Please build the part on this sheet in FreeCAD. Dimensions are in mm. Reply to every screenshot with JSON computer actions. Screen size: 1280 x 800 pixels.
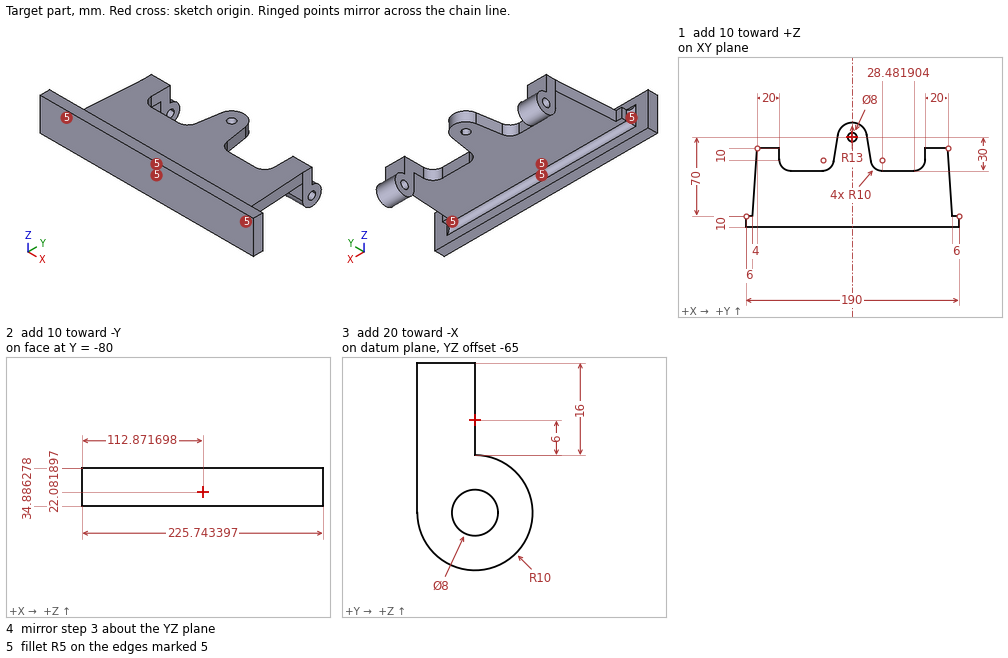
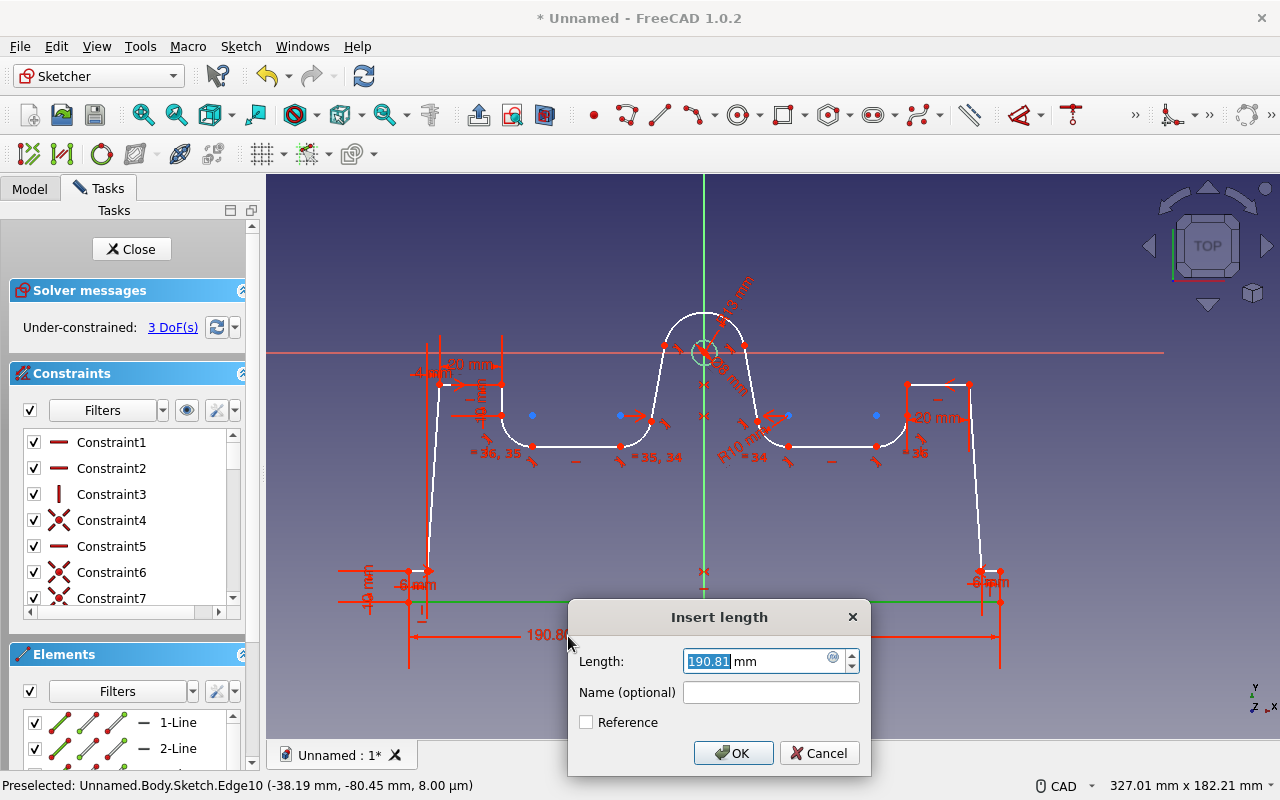
{"action": "type", "text": "190"}
{"action": "key", "text": "Return"}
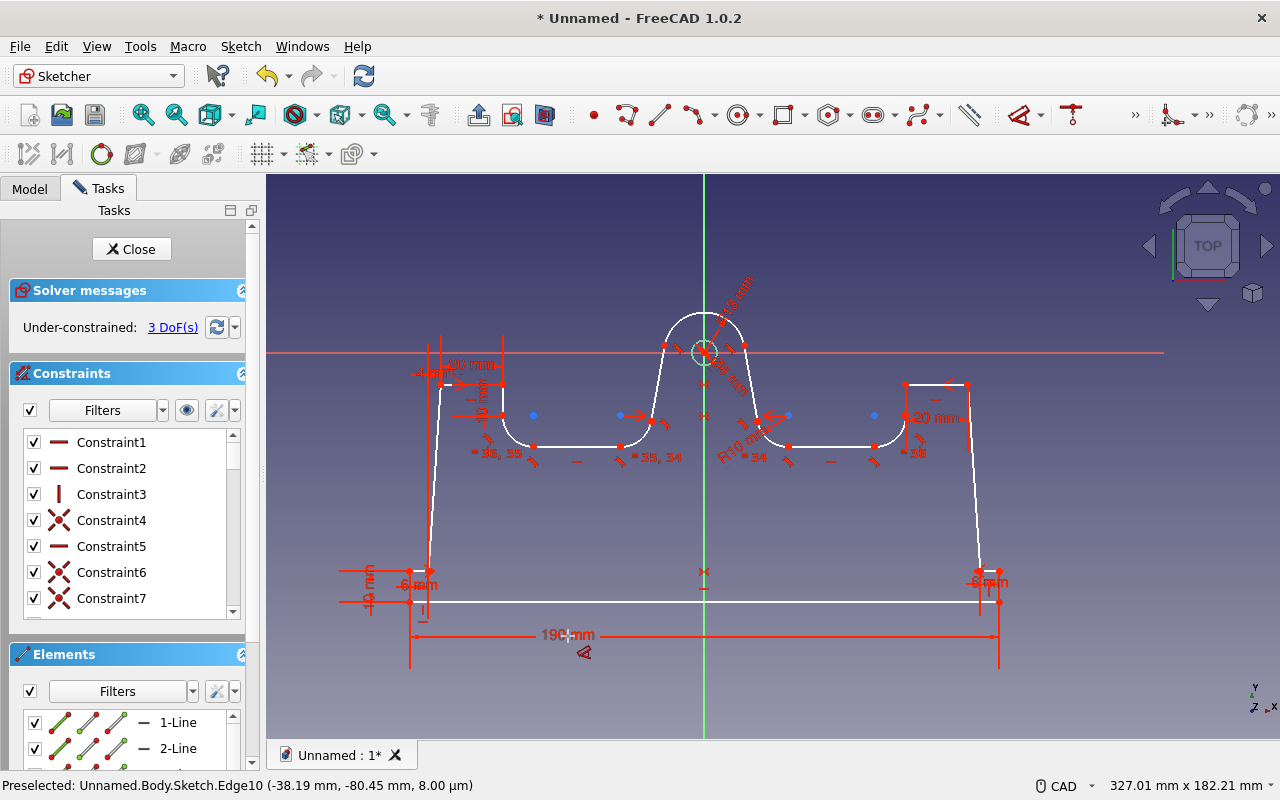
{"action": "left_click", "coordinate": [875, 447]}
{"action": "left_click", "coordinate": [909, 367]}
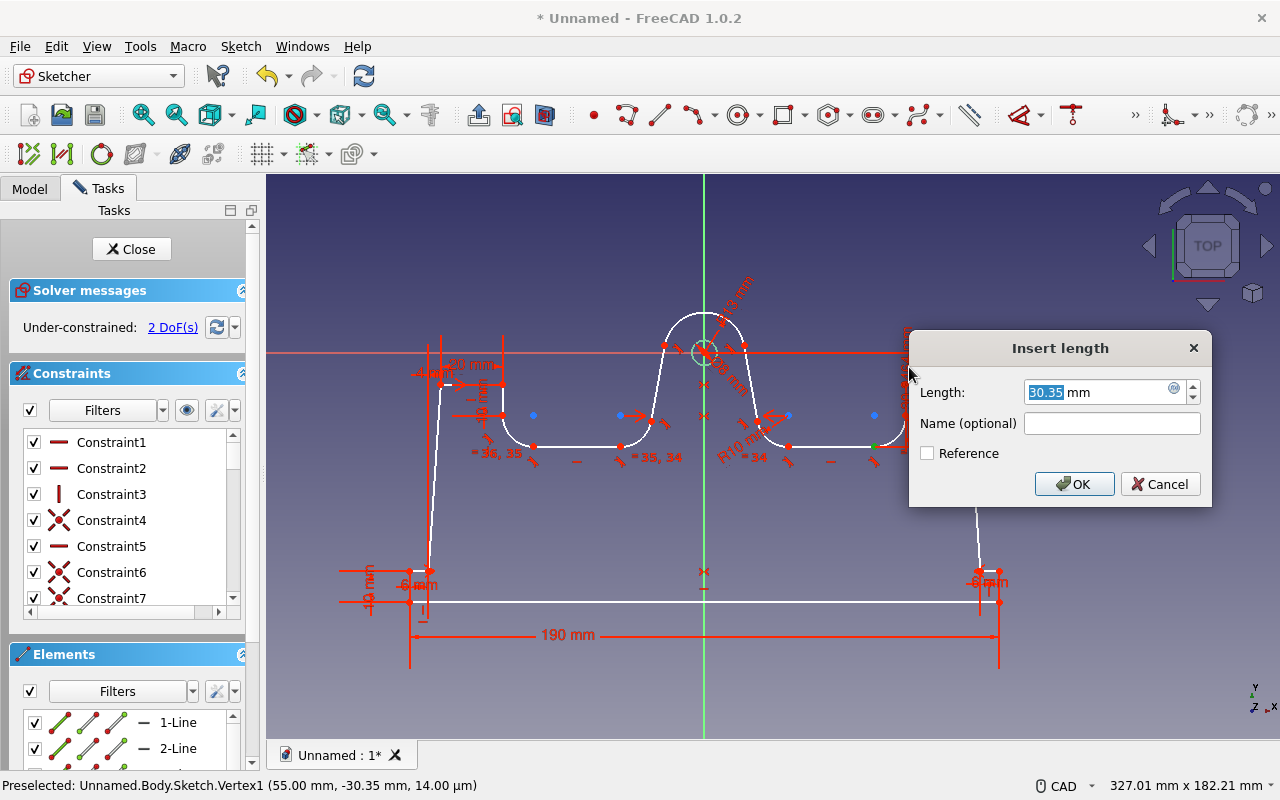
{"action": "type", "text": "30"}
{"action": "key", "text": "Return"}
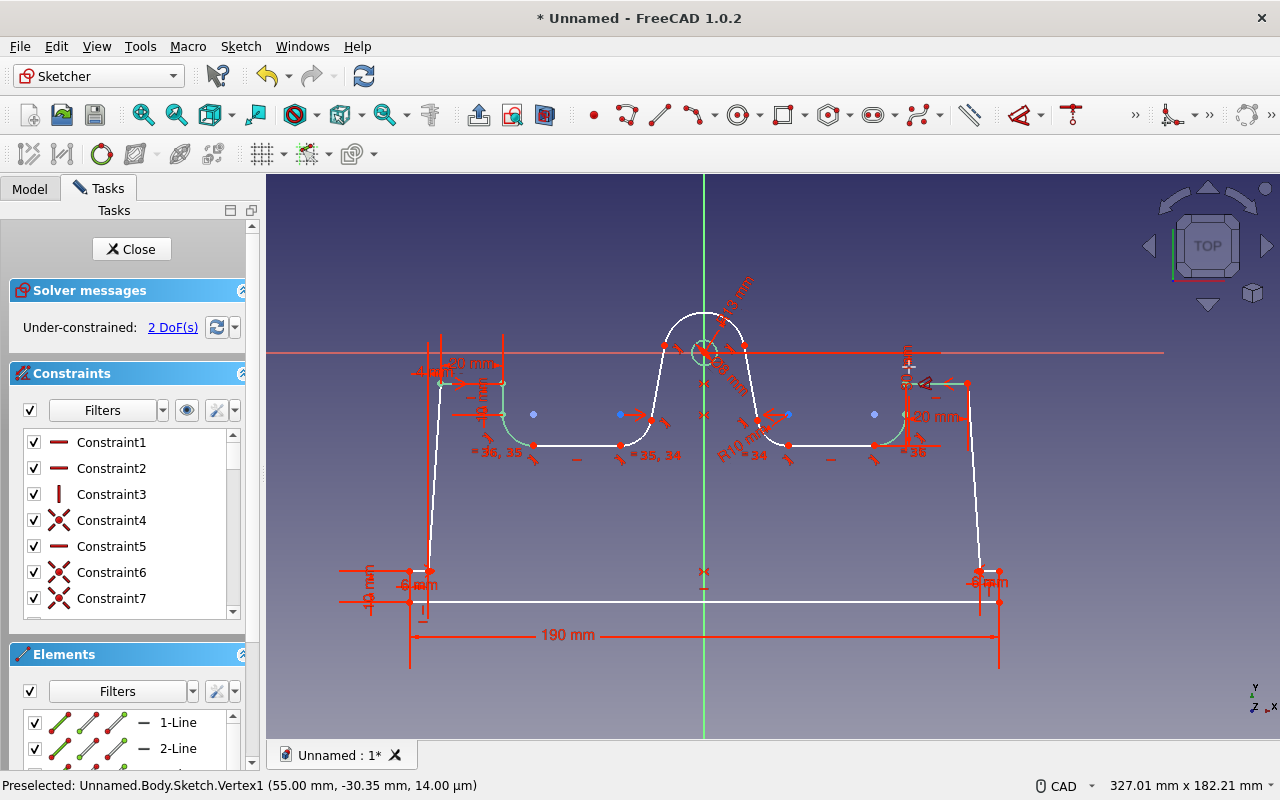
{"action": "left_click", "coordinate": [428, 571]}
{"action": "left_click", "coordinate": [394, 462]}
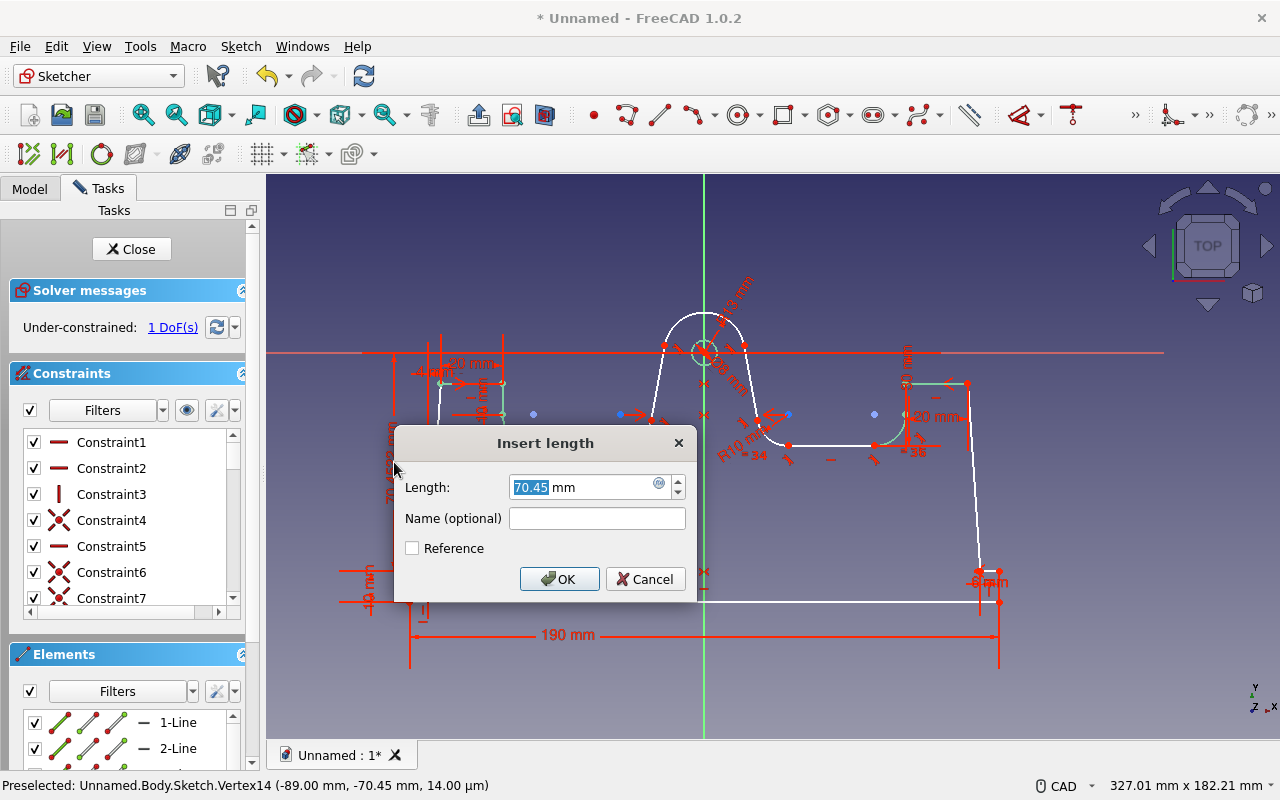
{"action": "type", "text": "70"}
{"action": "key", "text": "Return"}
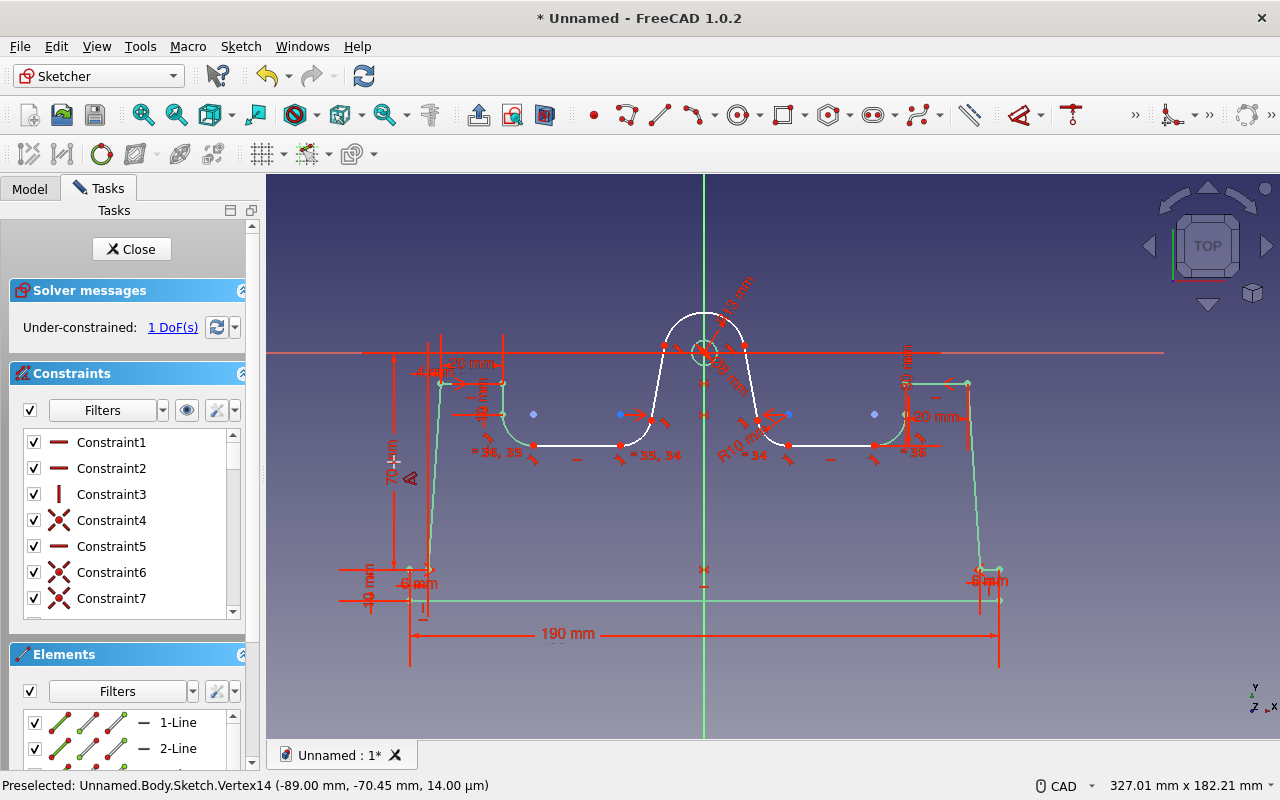
{"action": "left_click", "coordinate": [849, 446]}
{"action": "left_click", "coordinate": [832, 412]}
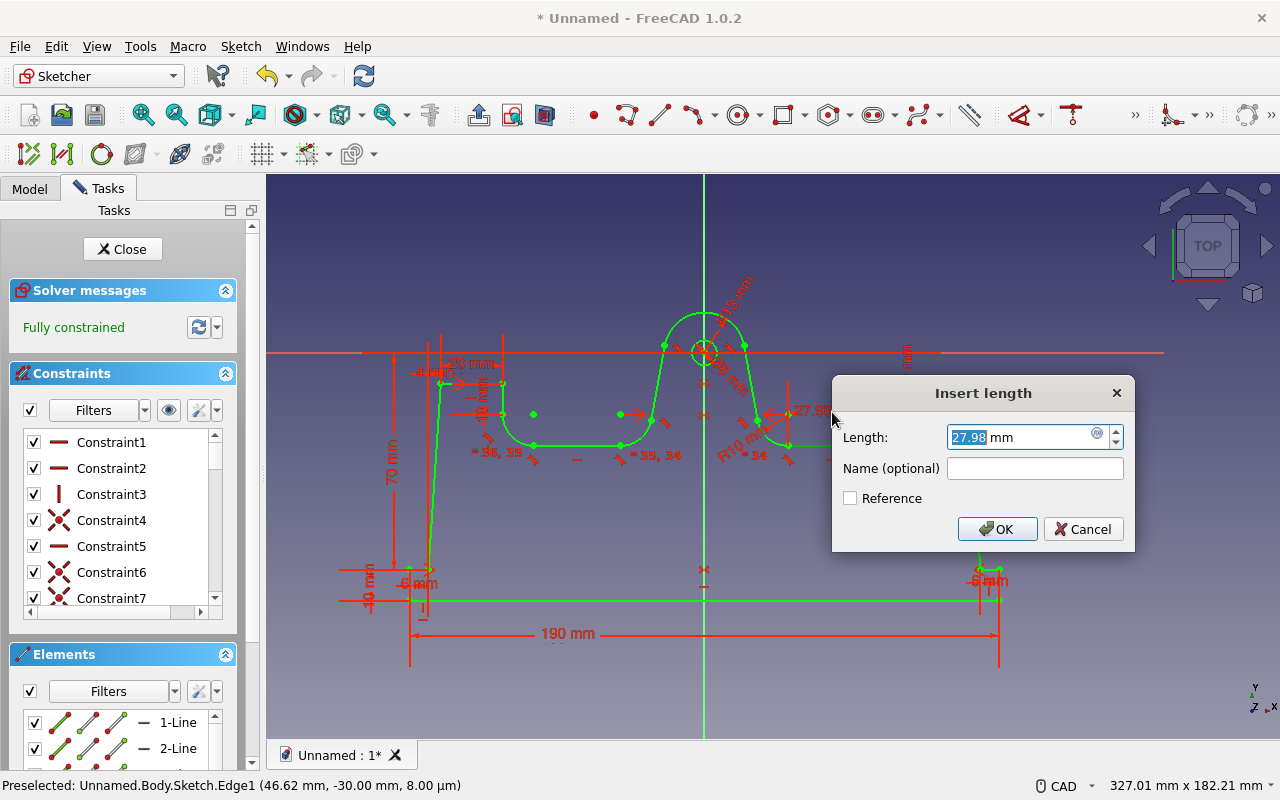
{"action": "type", "text": "28.481904"}
{"action": "key", "text": "Return"}
{"action": "key", "text": "Escape"}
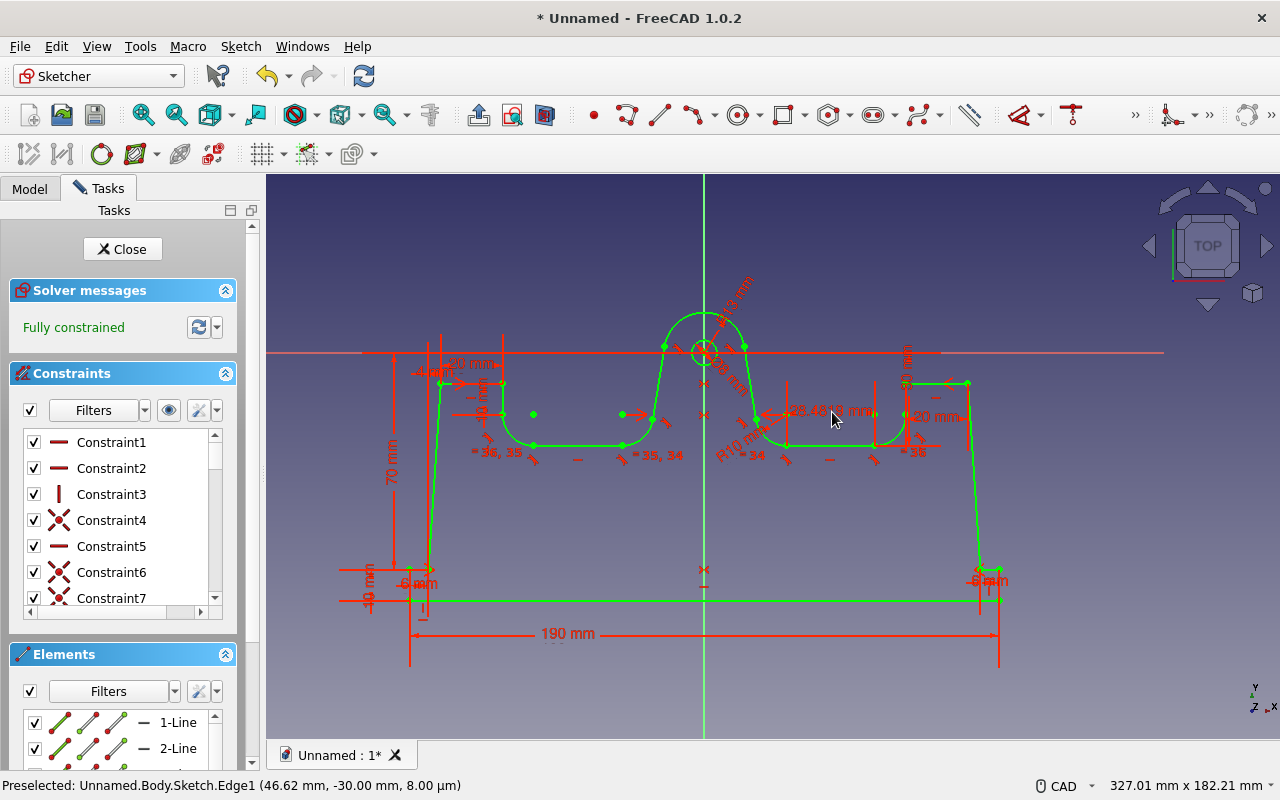
{"action": "left_click", "coordinate": [123, 249]}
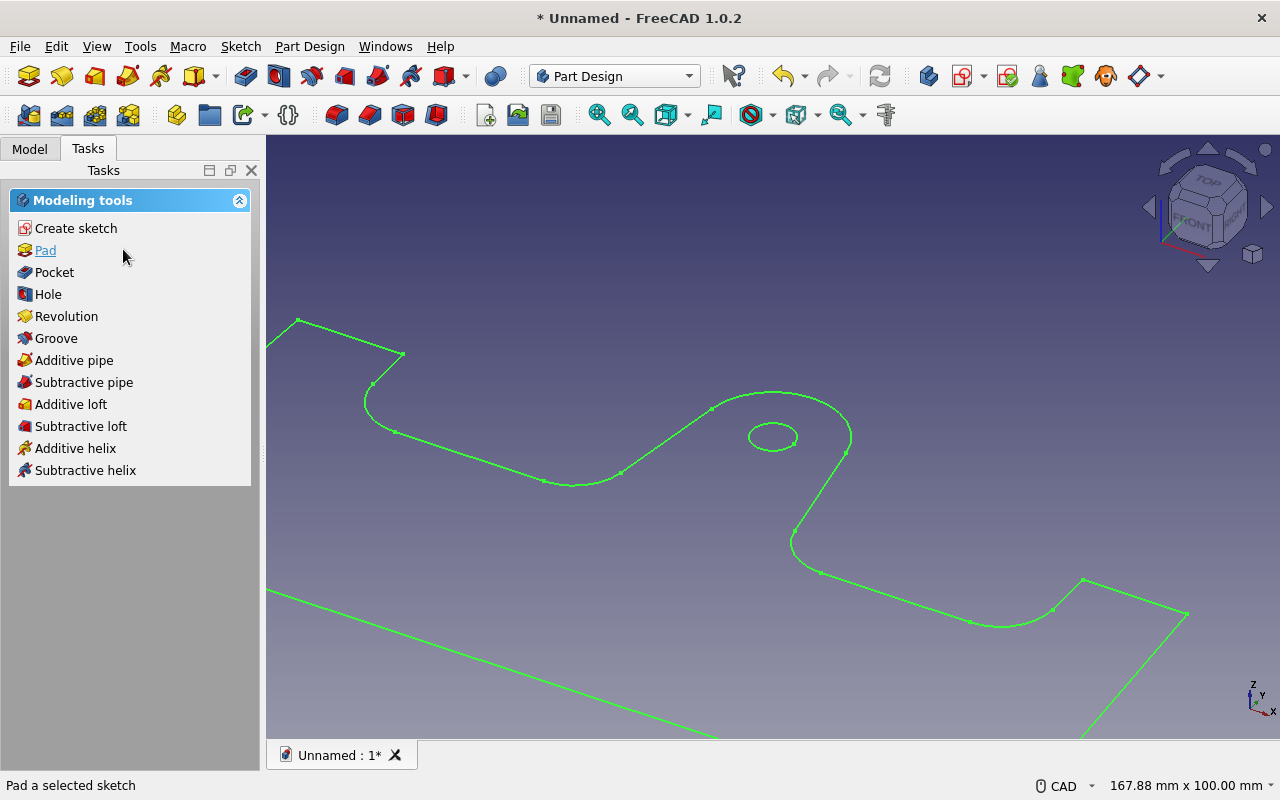
{"action": "left_click", "coordinate": [29, 76]}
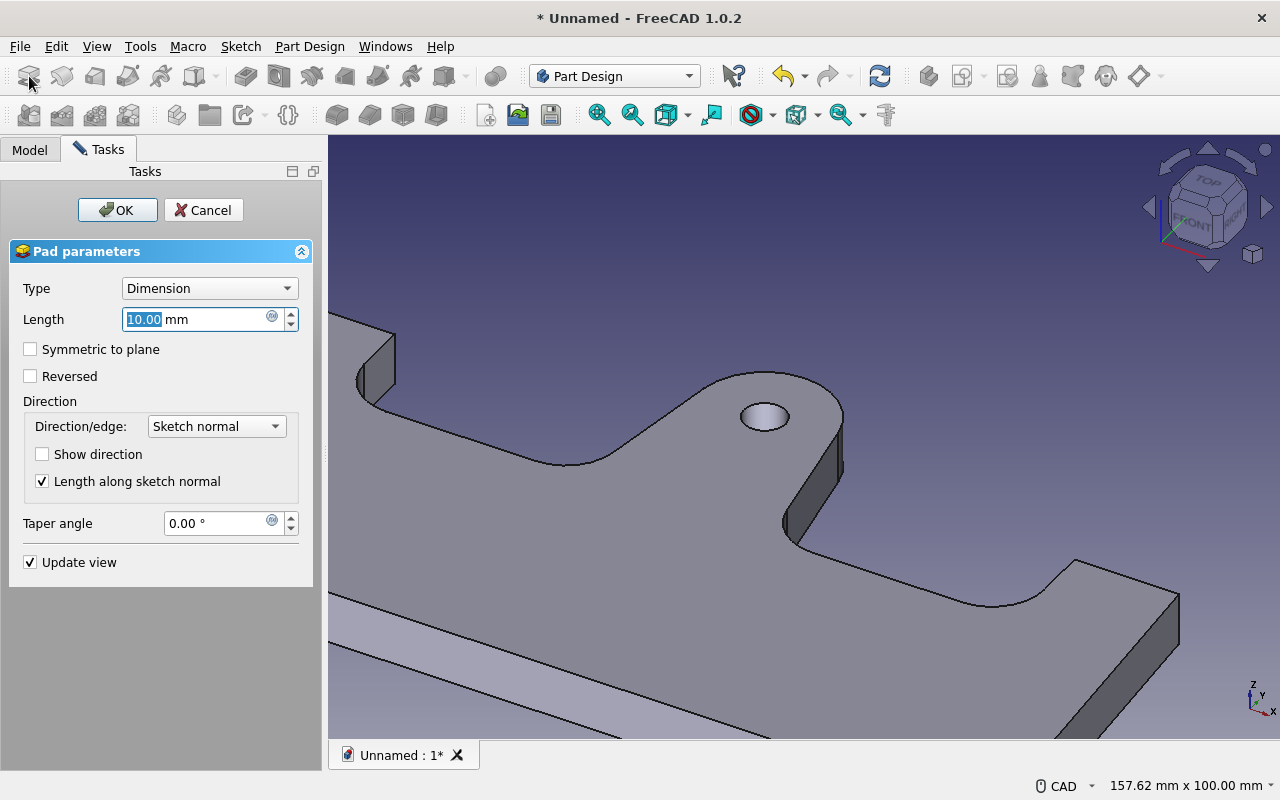
{"action": "type", "text": "10"}
{"action": "key", "text": "Tab"}